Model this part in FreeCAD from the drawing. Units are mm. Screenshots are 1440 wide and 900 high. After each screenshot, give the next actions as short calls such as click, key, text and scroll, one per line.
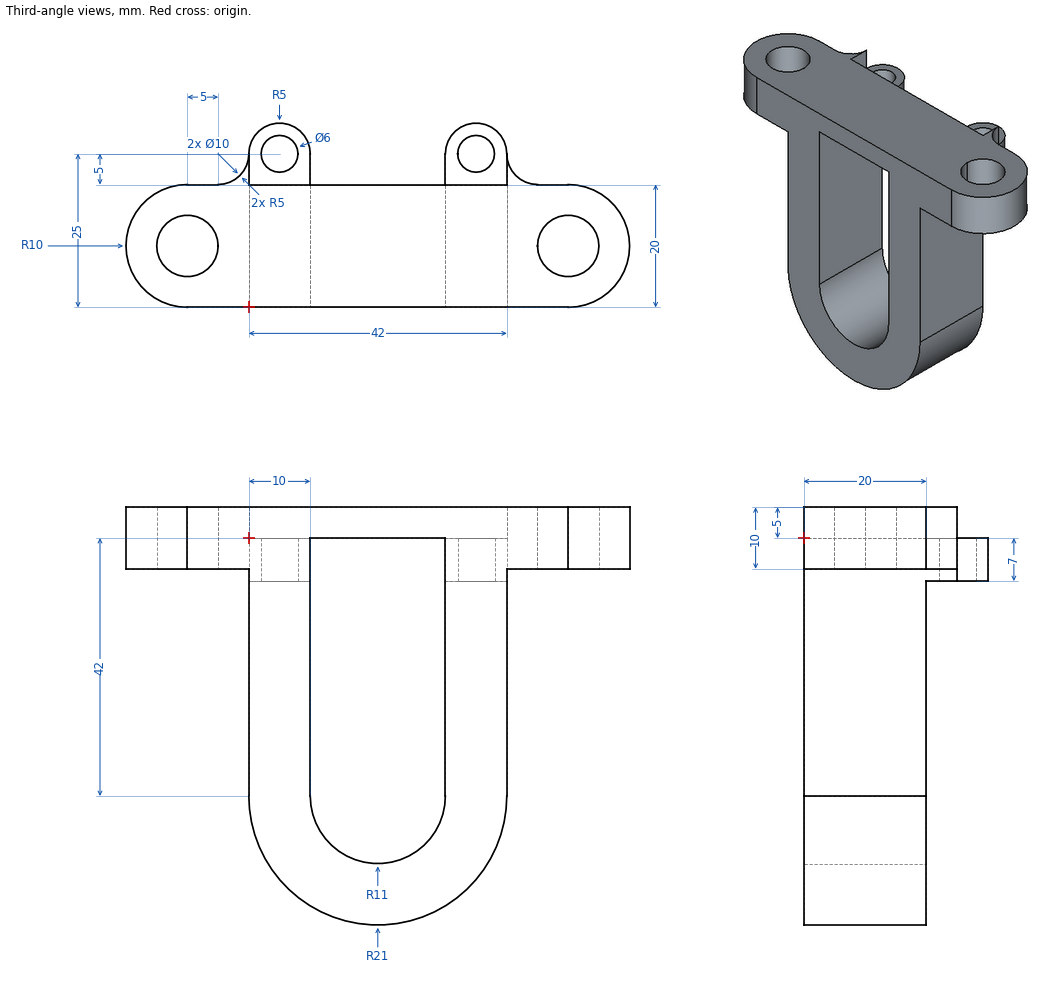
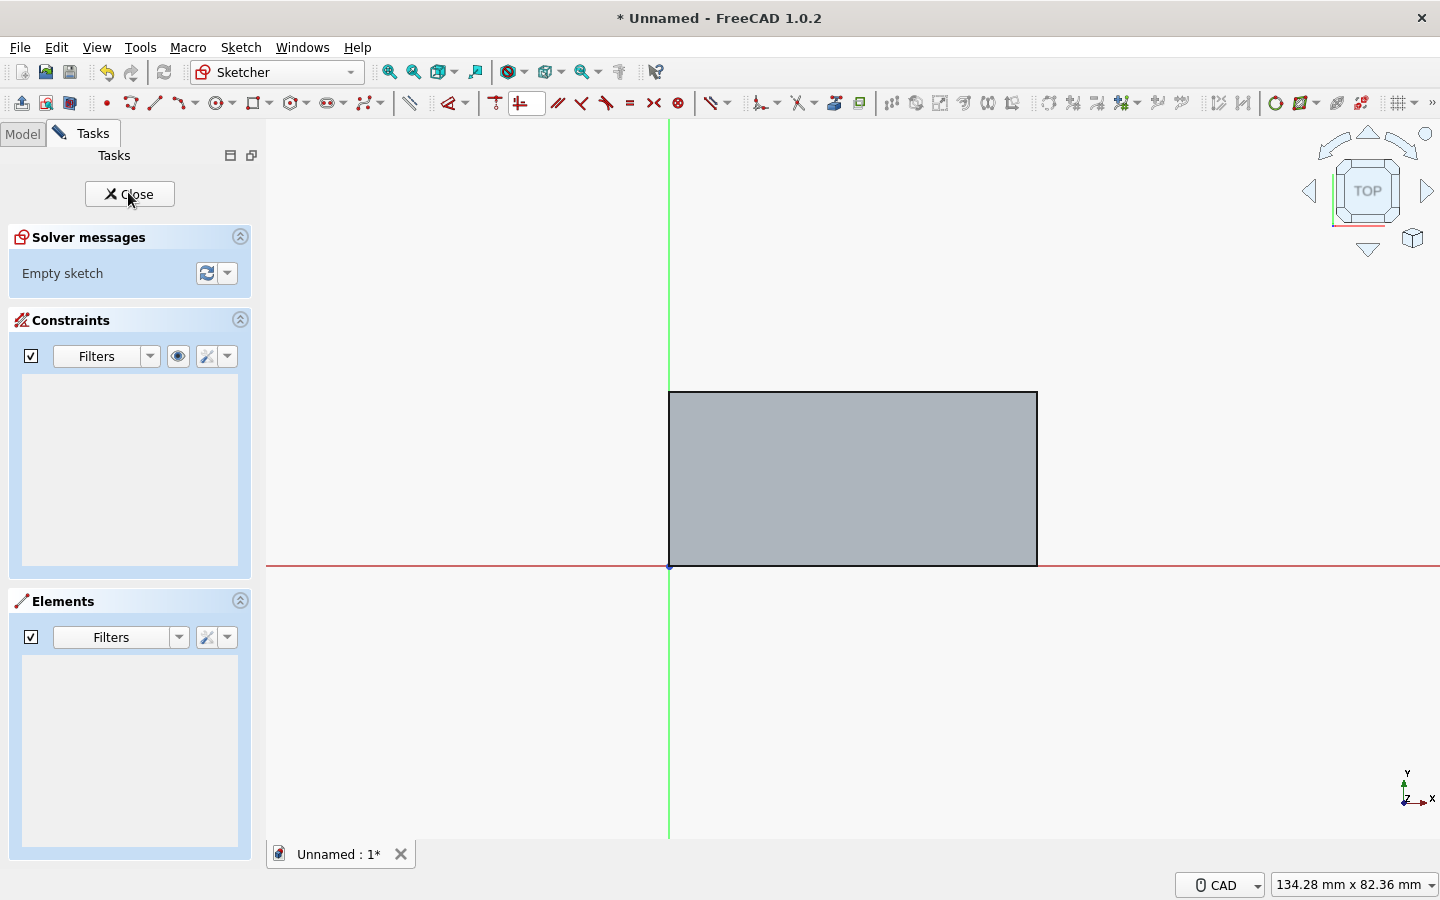
click(70, 104)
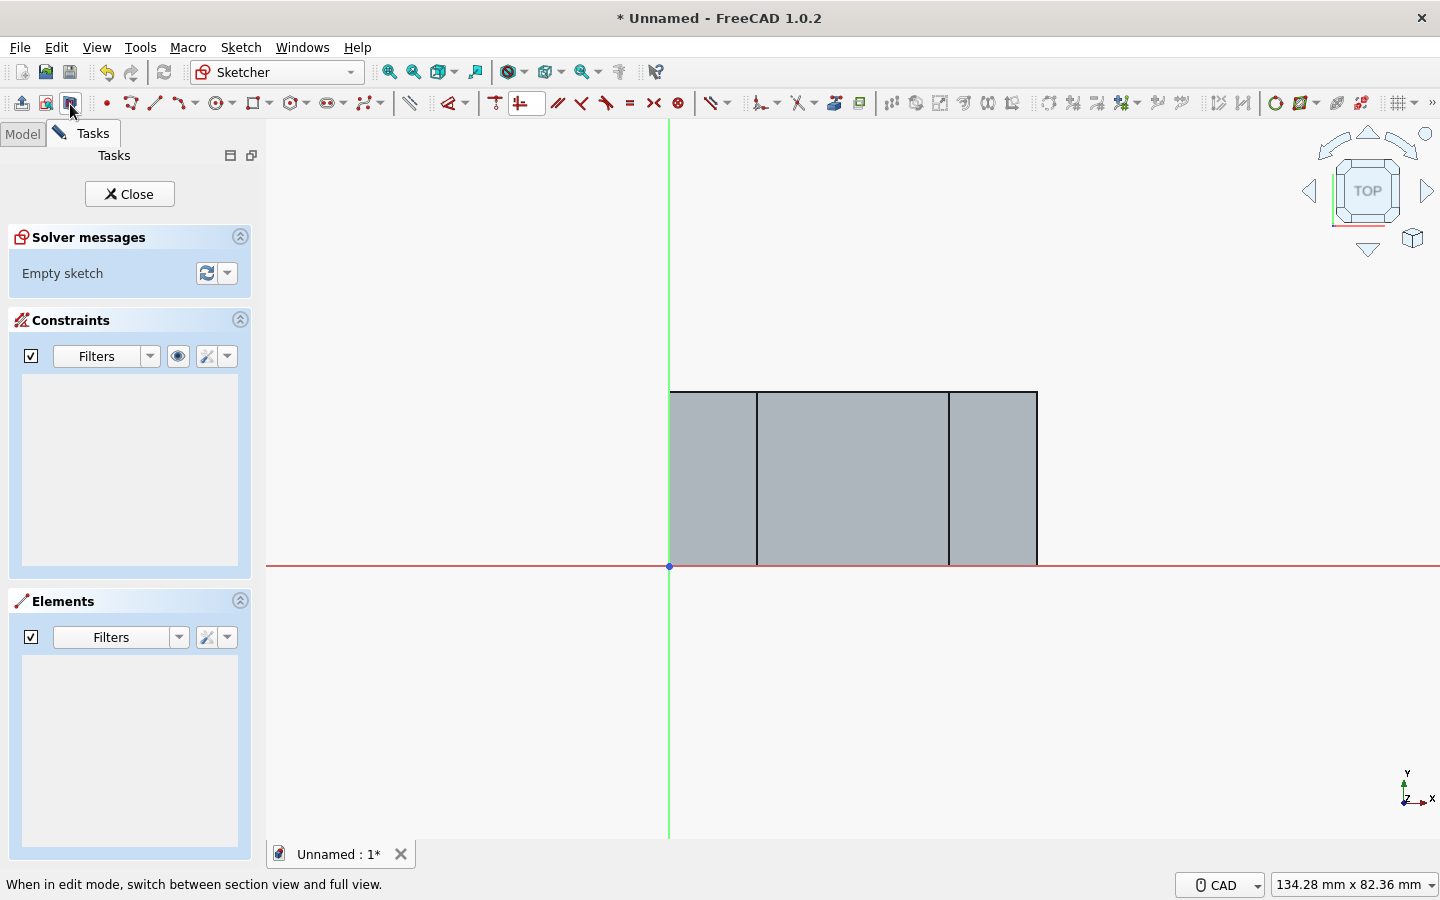
scroll(695, 315, up, 8)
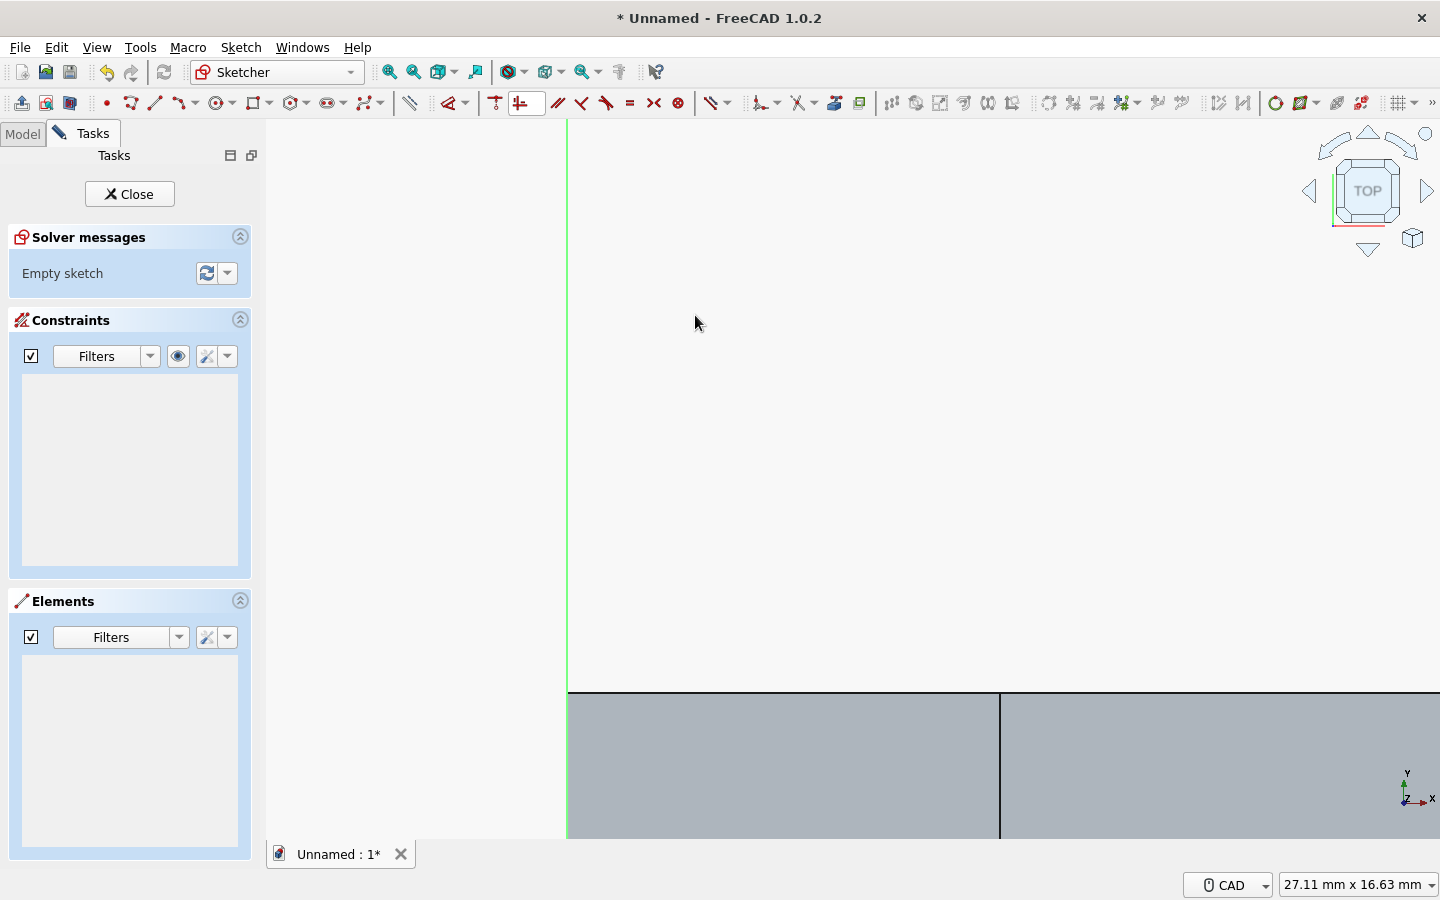
click(132, 104)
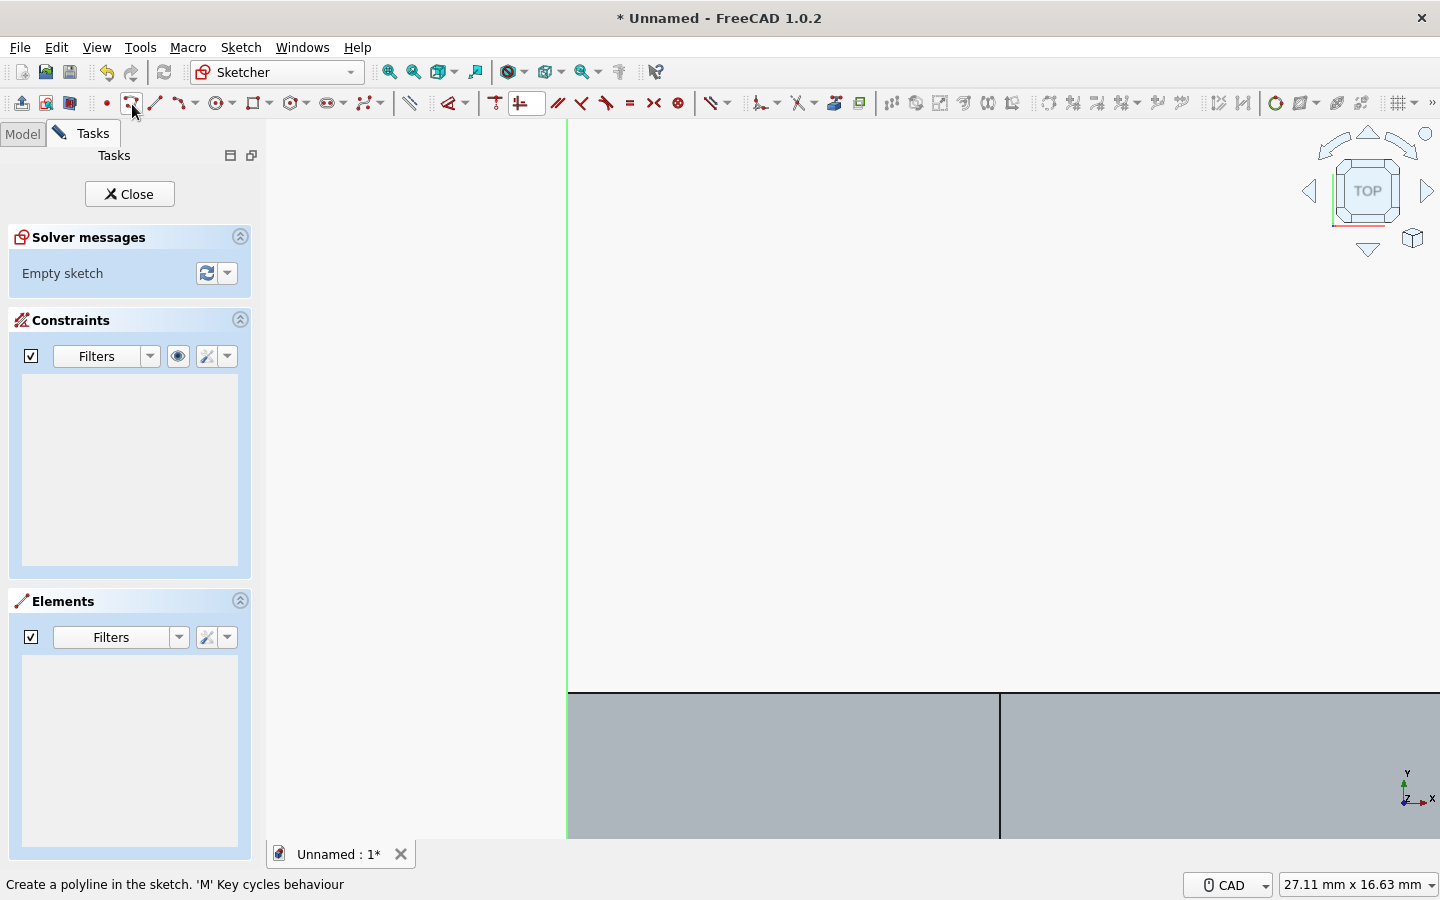
click(567, 477)
click(576, 693)
click(1000, 693)
click(1000, 477)
right_click(1000, 477)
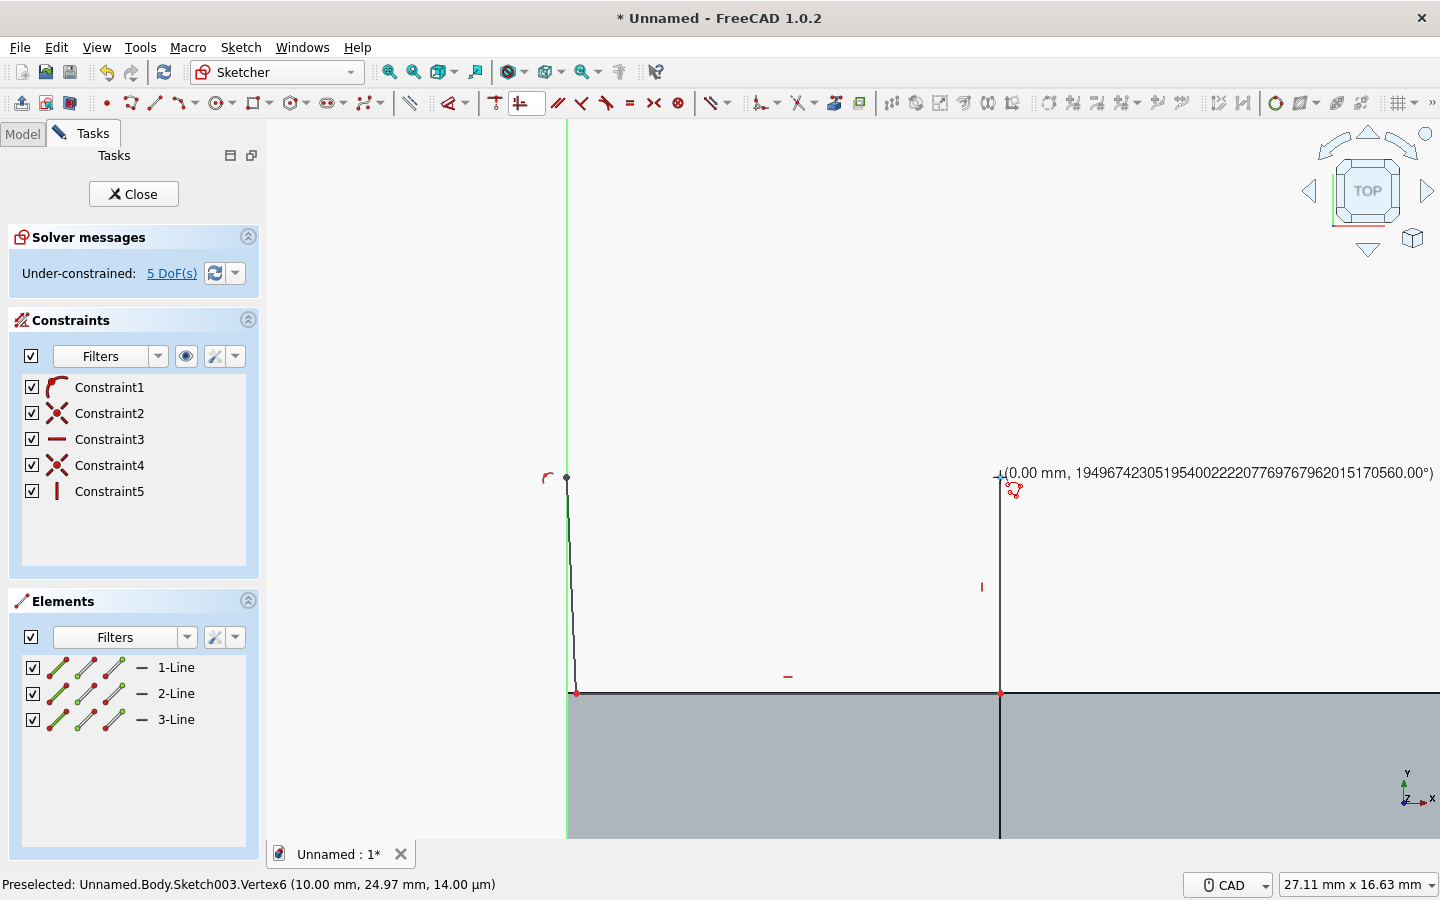
click(180, 104)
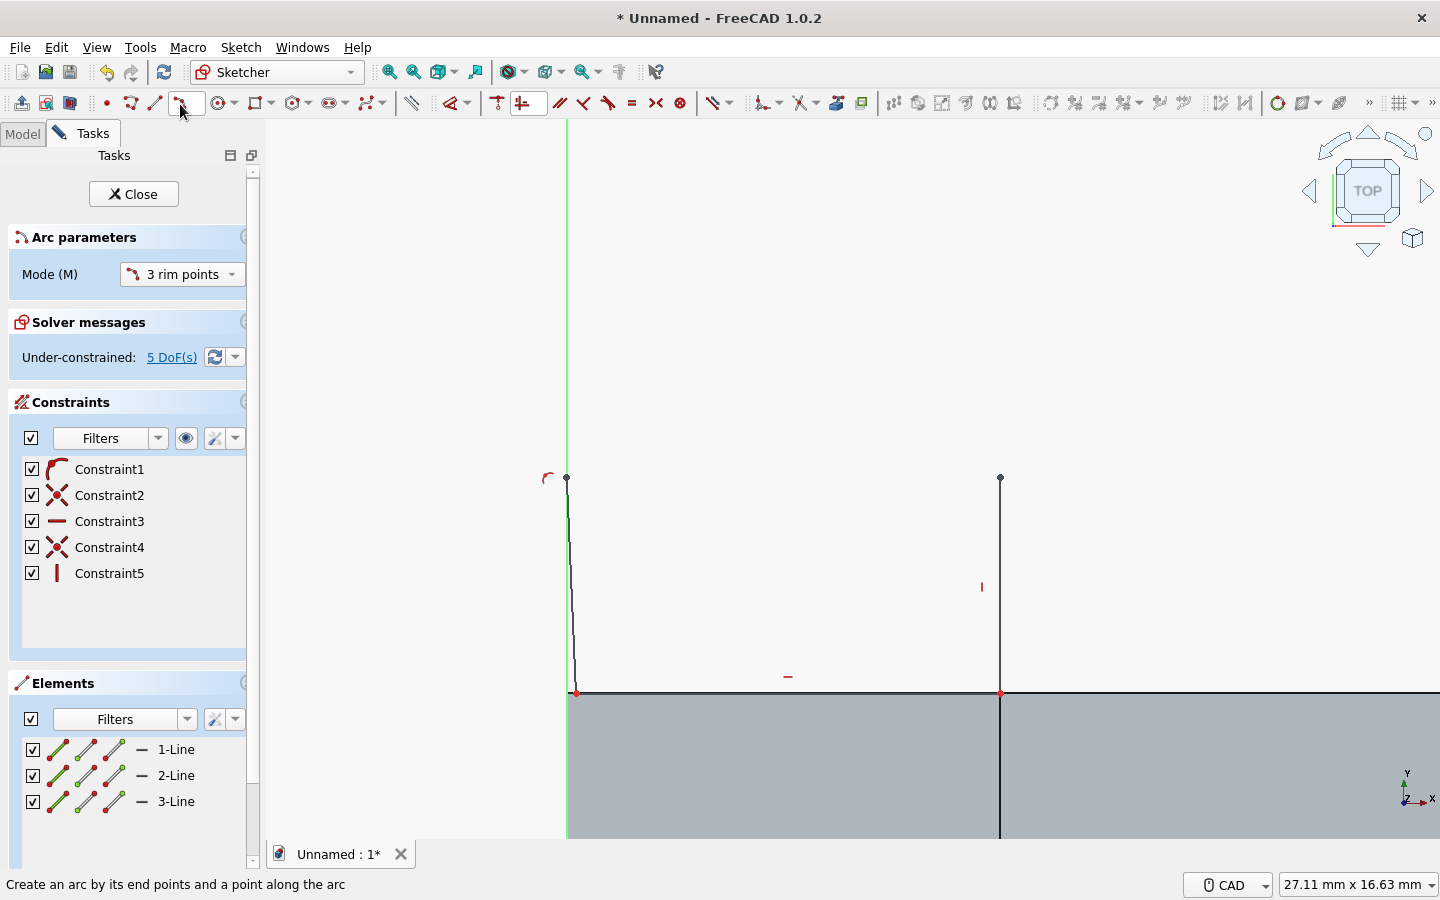
click(1000, 478)
click(567, 478)
click(783, 260)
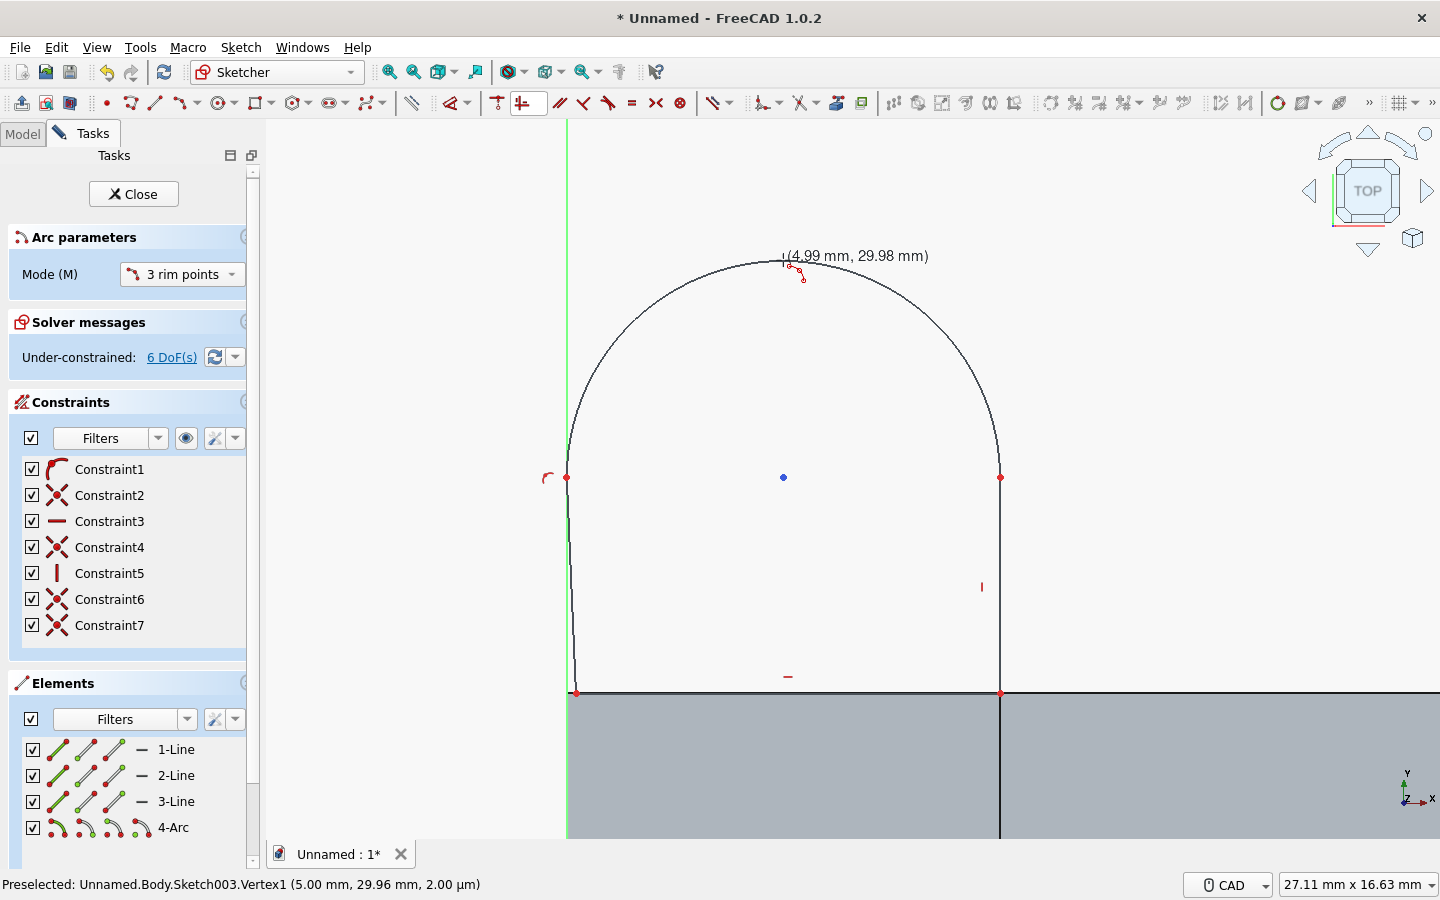
click(218, 104)